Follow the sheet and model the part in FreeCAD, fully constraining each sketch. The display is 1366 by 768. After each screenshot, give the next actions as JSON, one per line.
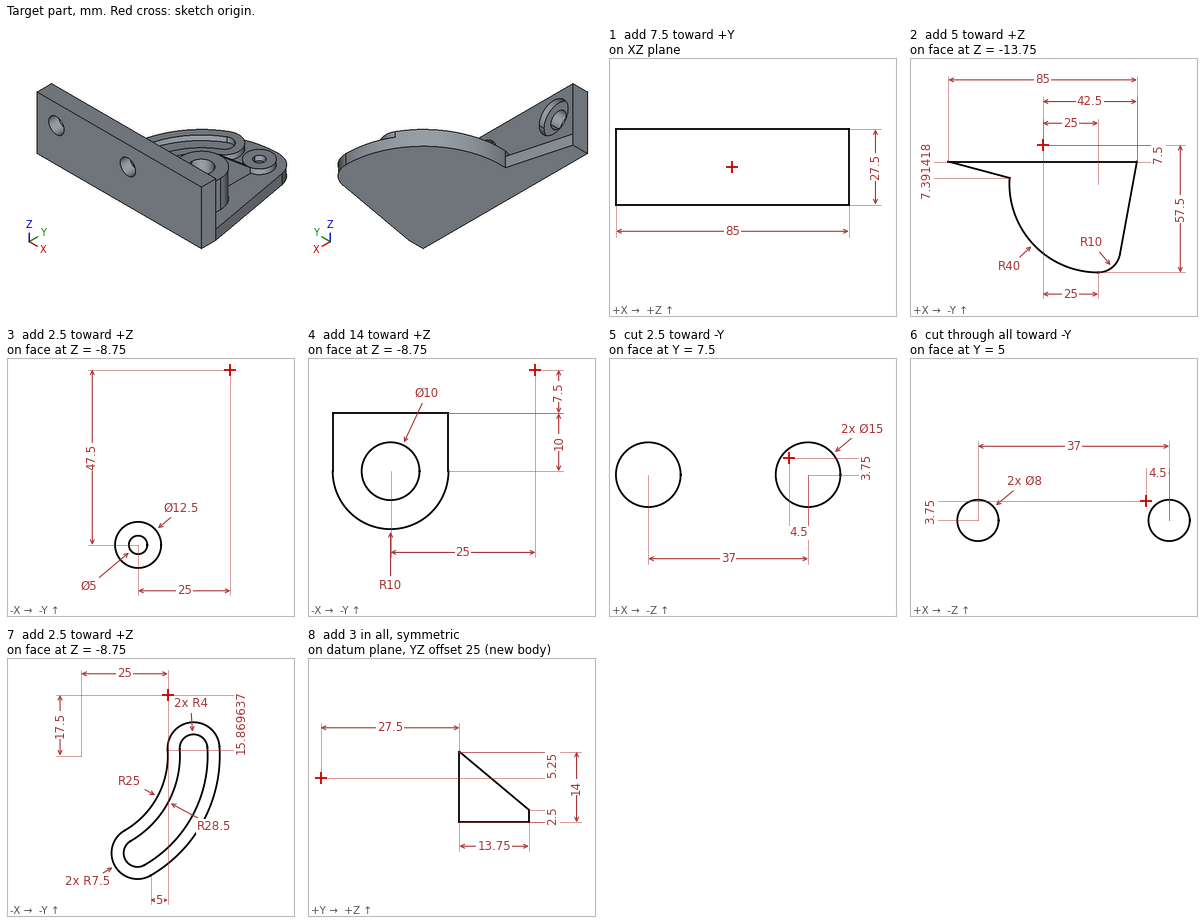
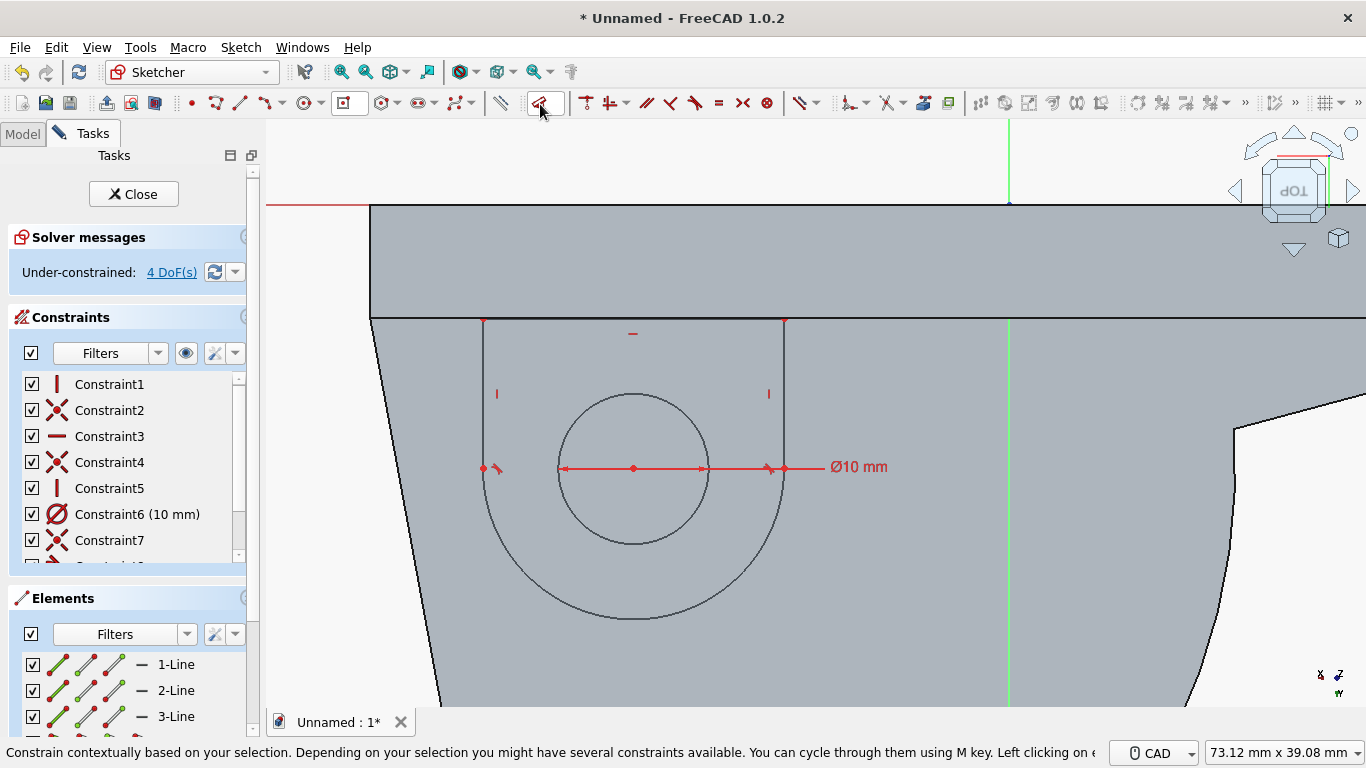
{"action": "left_click", "coordinate": [545, 591]}
{"action": "left_click", "coordinate": [526, 617]}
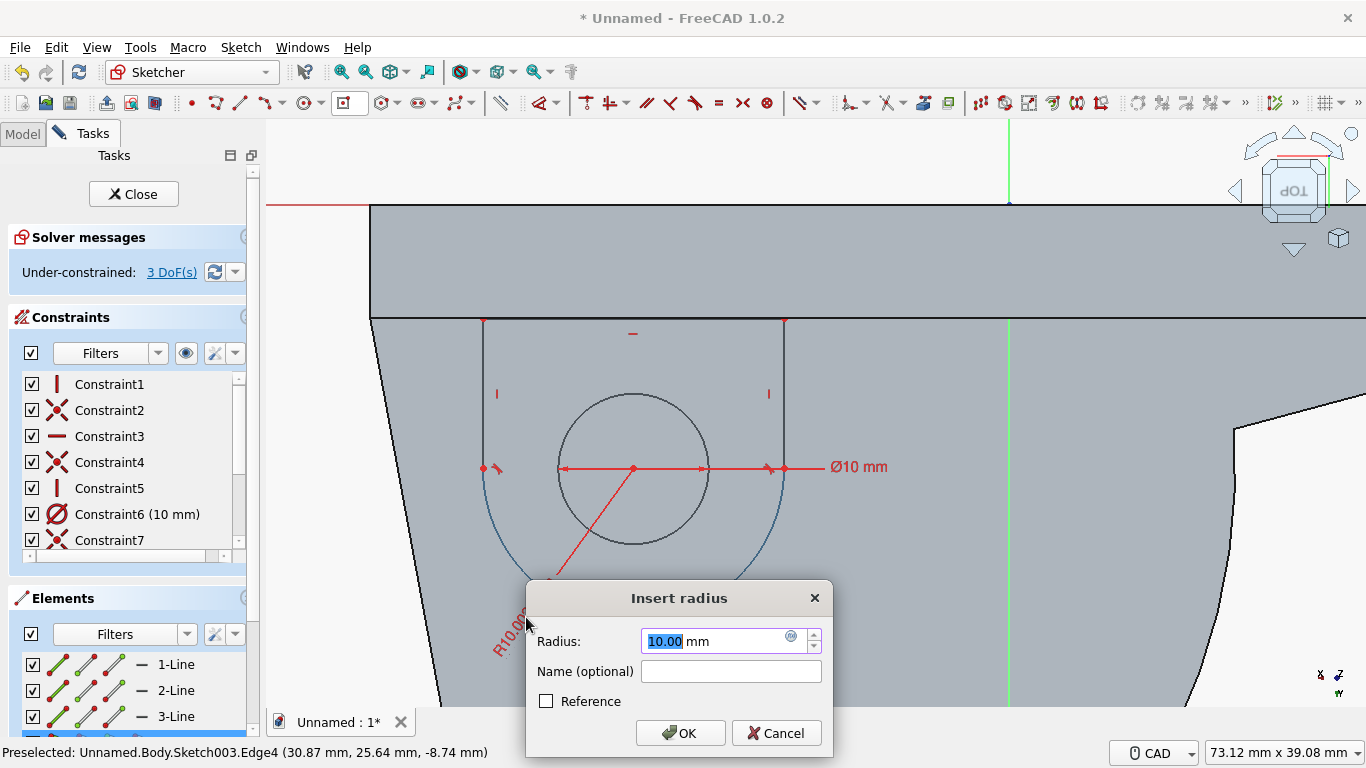
{"action": "type", "text": "10"}
{"action": "key", "text": "Return"}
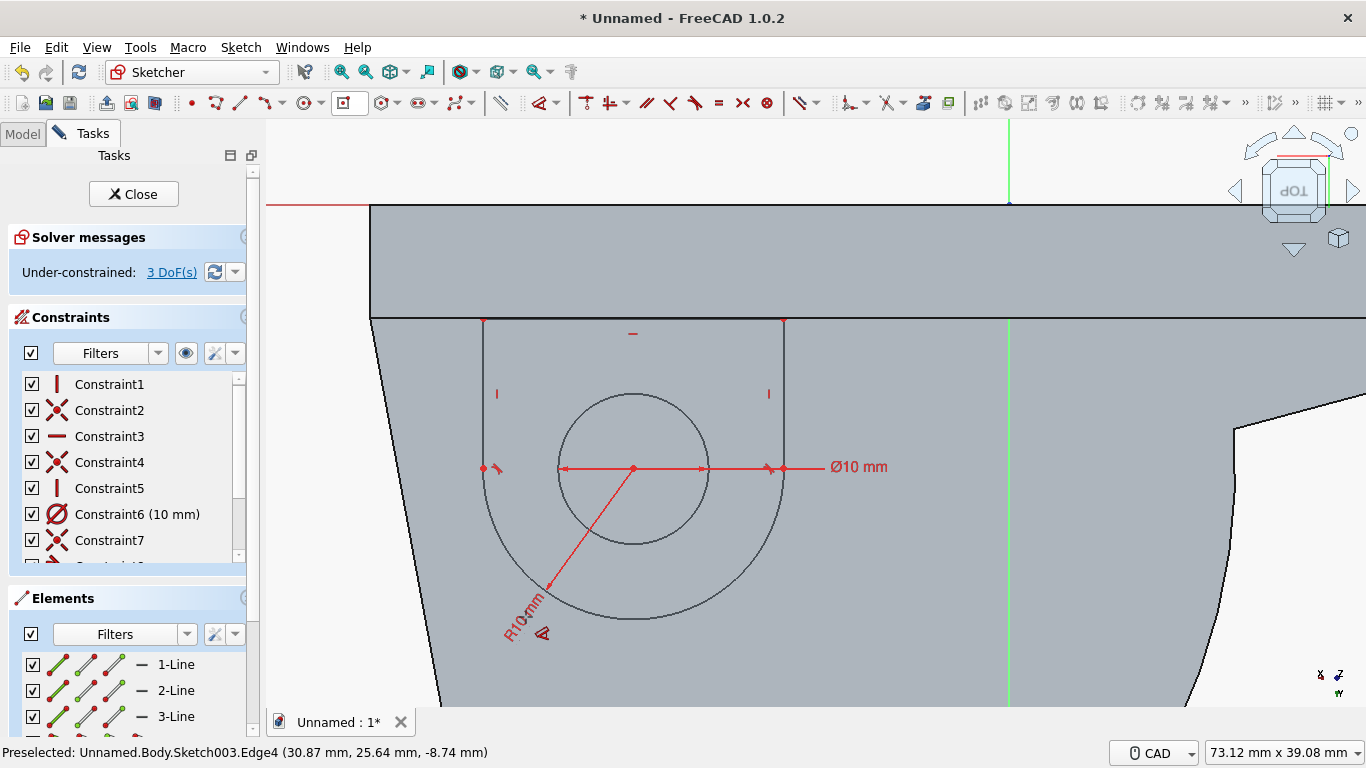
{"action": "left_click", "coordinate": [784, 424]}
{"action": "left_click", "coordinate": [818, 394]}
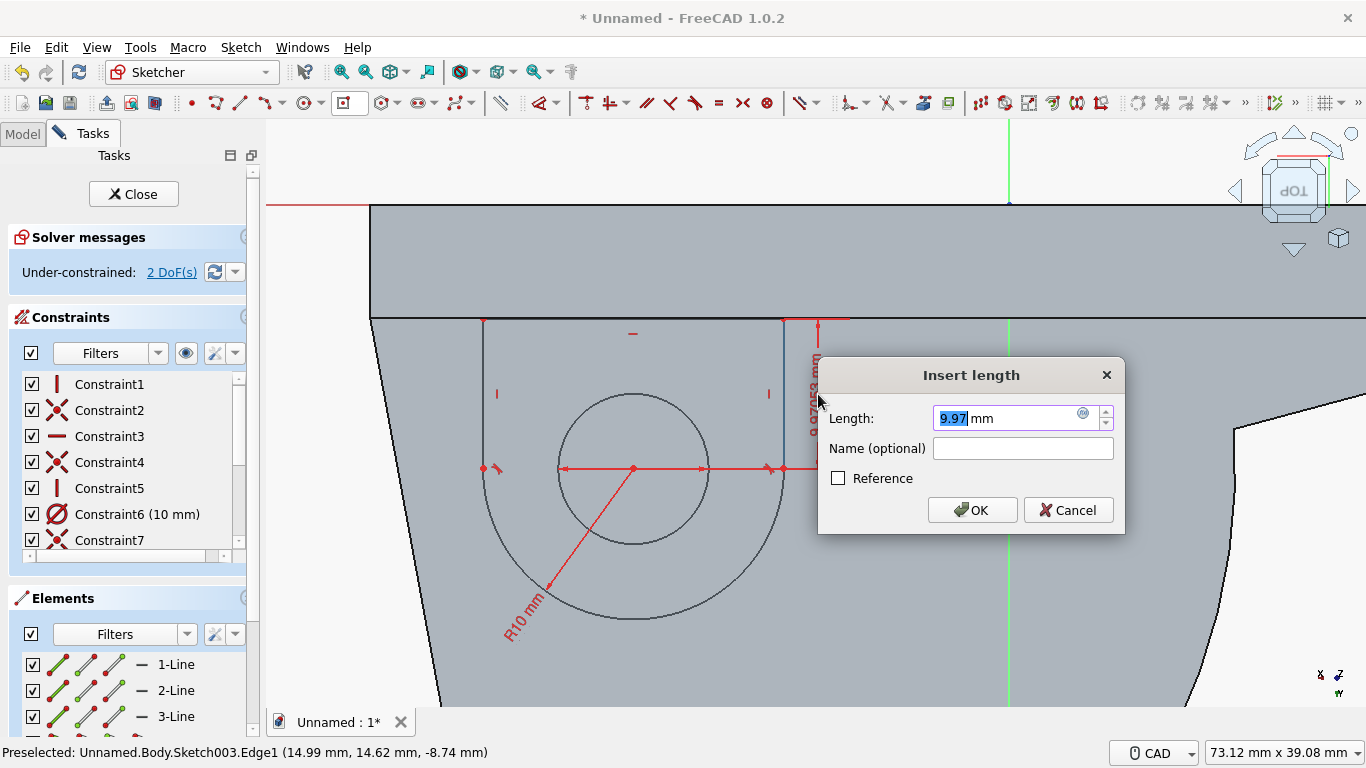
{"action": "type", "text": "10"}
{"action": "key", "text": "Return"}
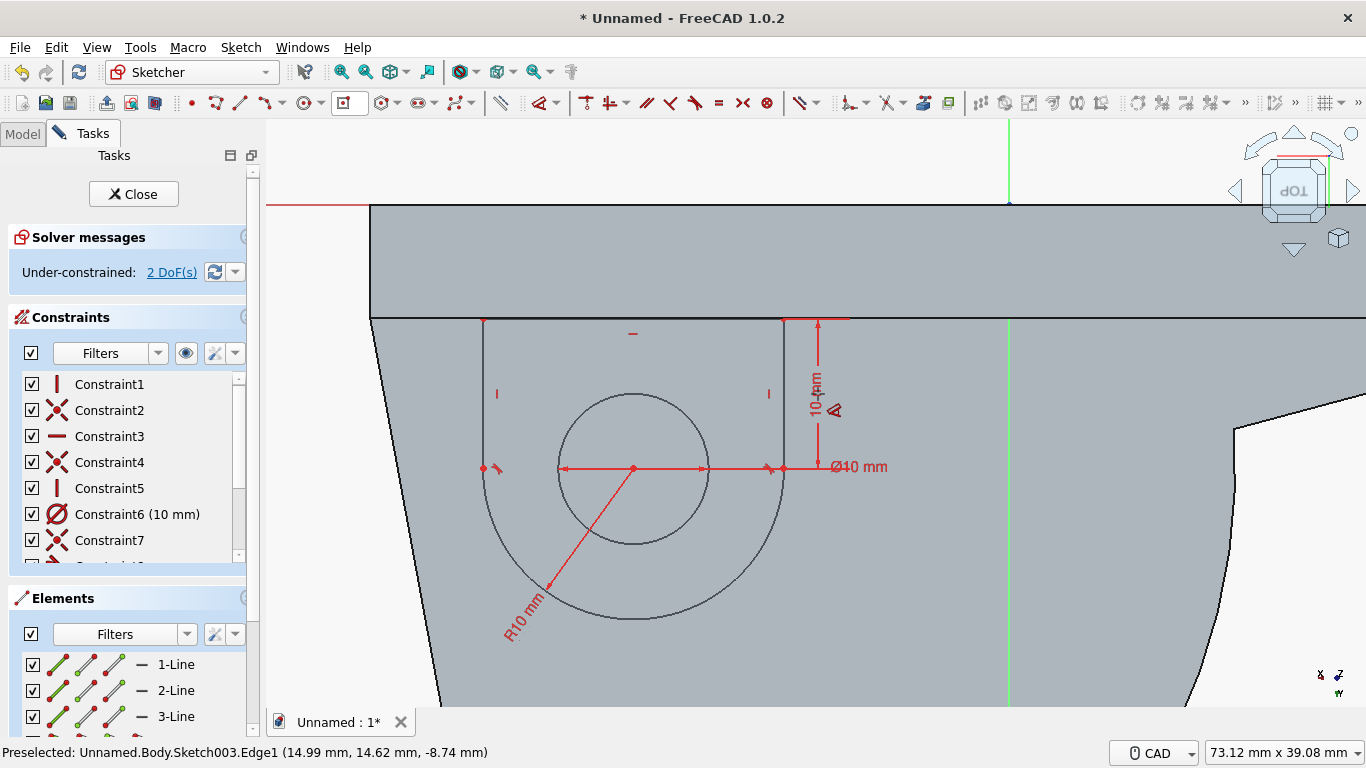
{"action": "left_click", "coordinate": [634, 469]}
{"action": "left_click", "coordinate": [821, 171]}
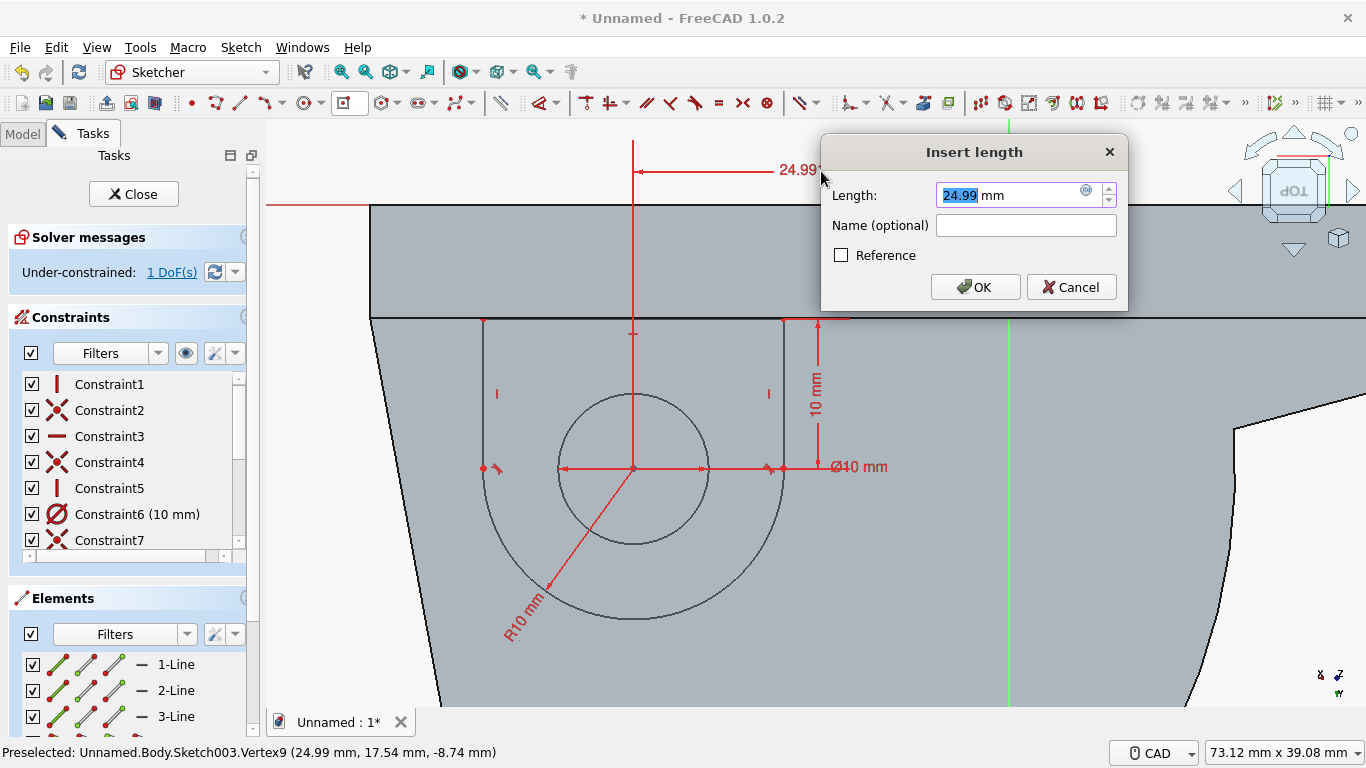
{"action": "type", "text": "25"}
{"action": "key", "text": "Return"}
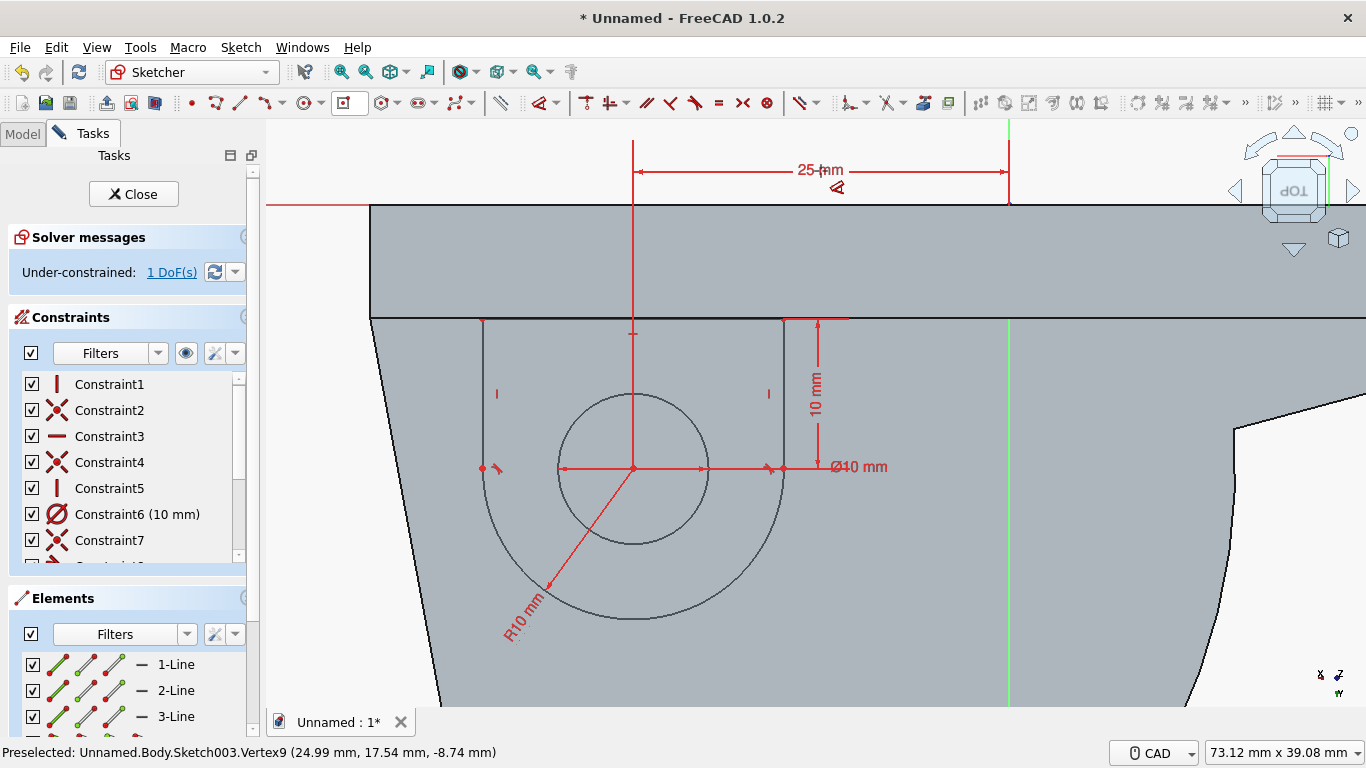
{"action": "left_click", "coordinate": [784, 319]}
{"action": "left_click", "coordinate": [1043, 262]}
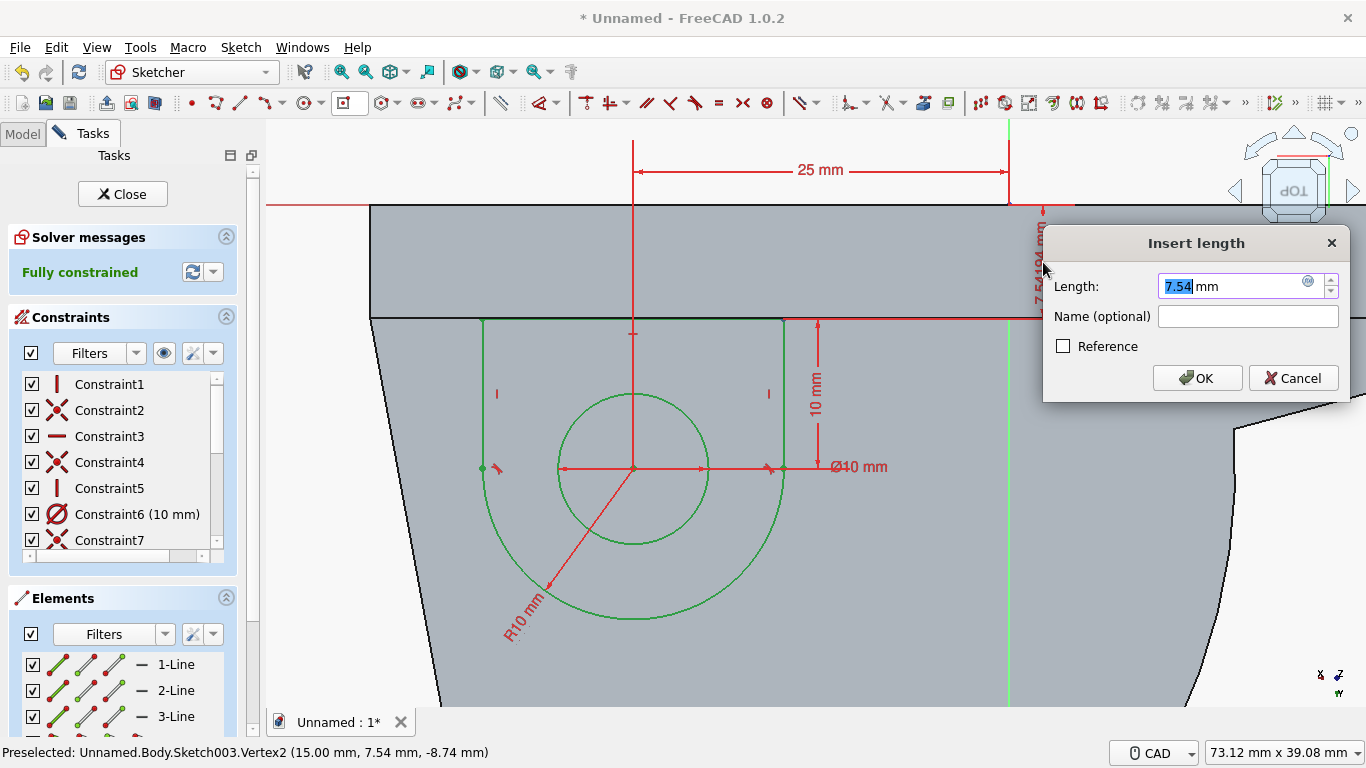
{"action": "type", "text": "7.5"}
{"action": "key", "text": "Return"}
{"action": "key", "text": "Escape"}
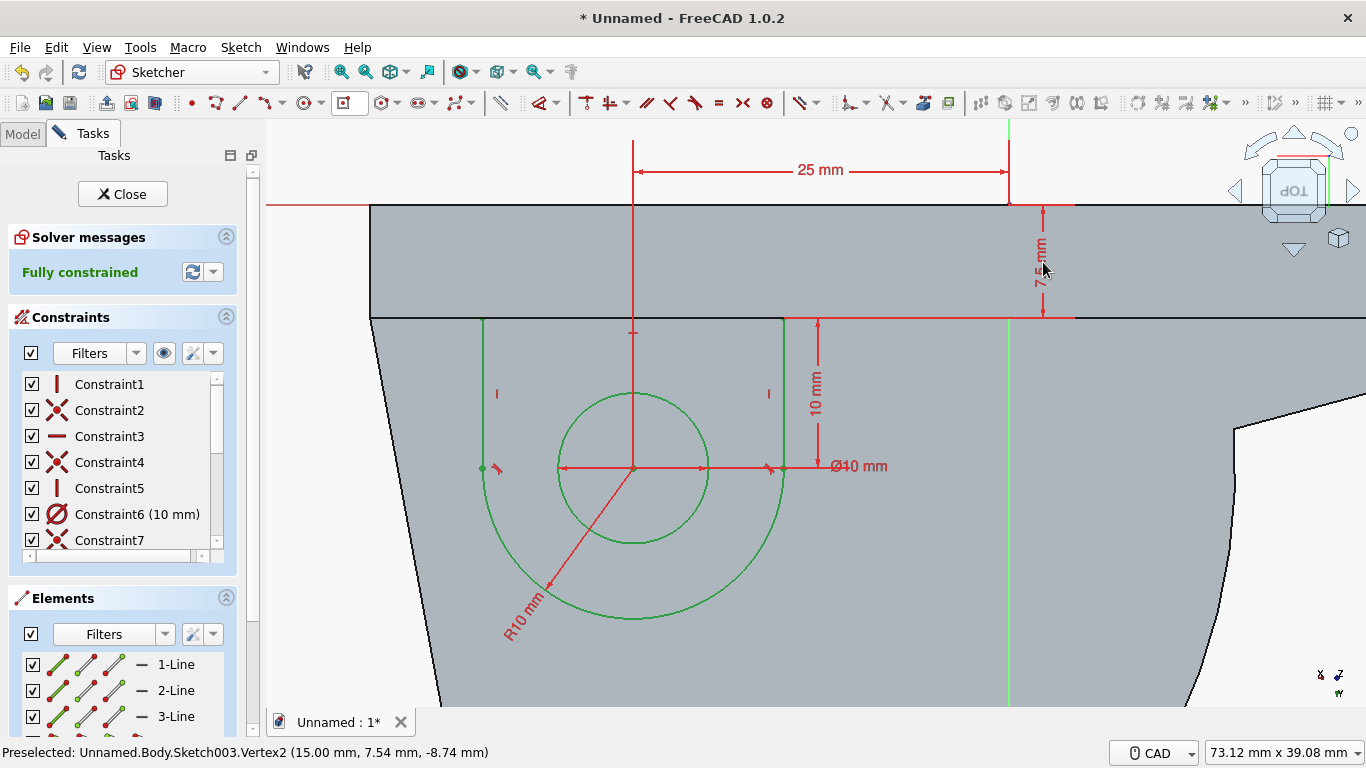
{"action": "left_click", "coordinate": [123, 194]}